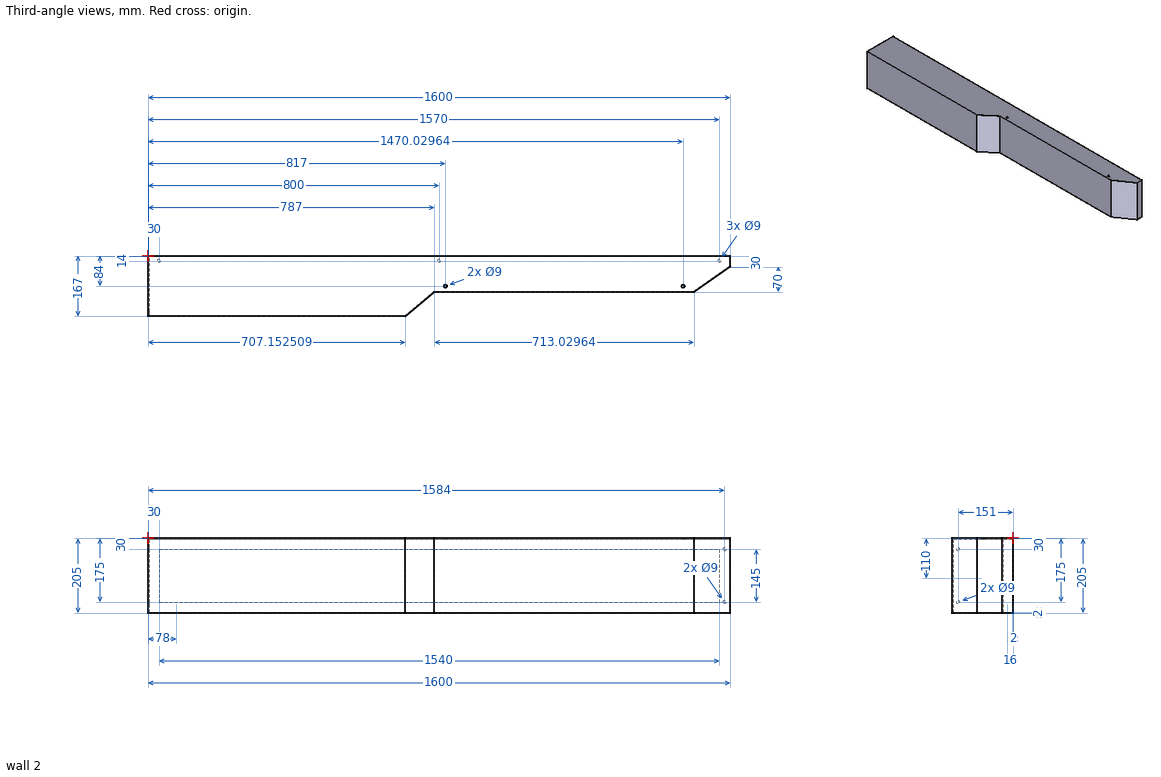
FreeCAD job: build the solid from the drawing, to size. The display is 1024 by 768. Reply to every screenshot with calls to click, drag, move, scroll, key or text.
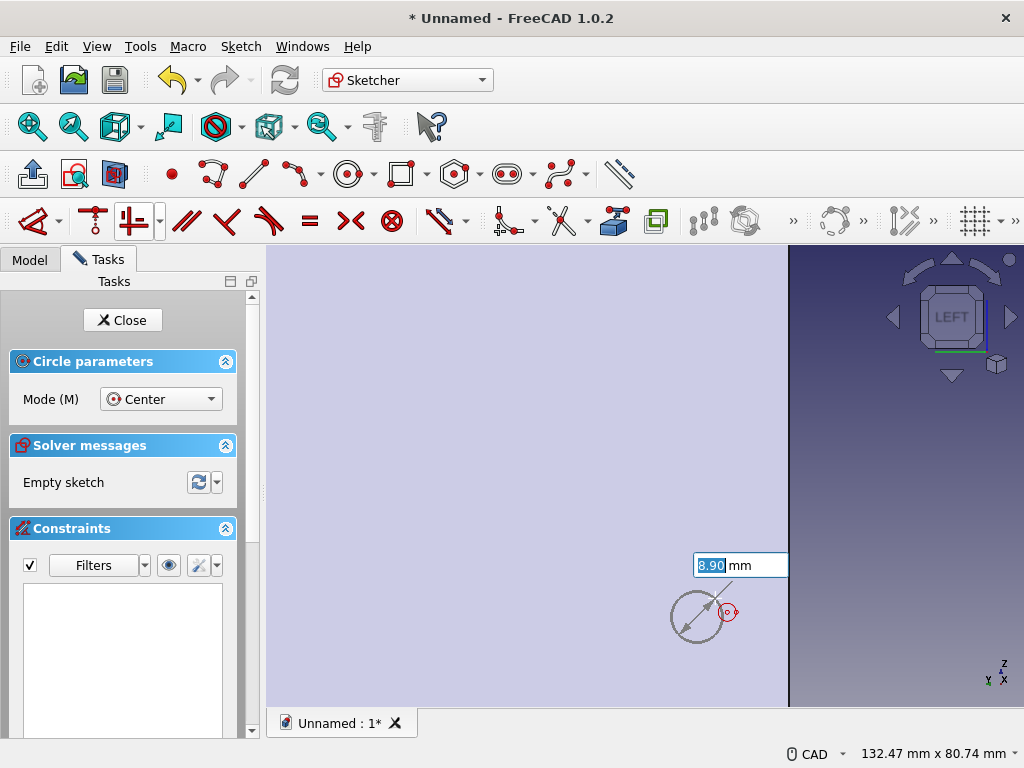
text(9)
key(Return)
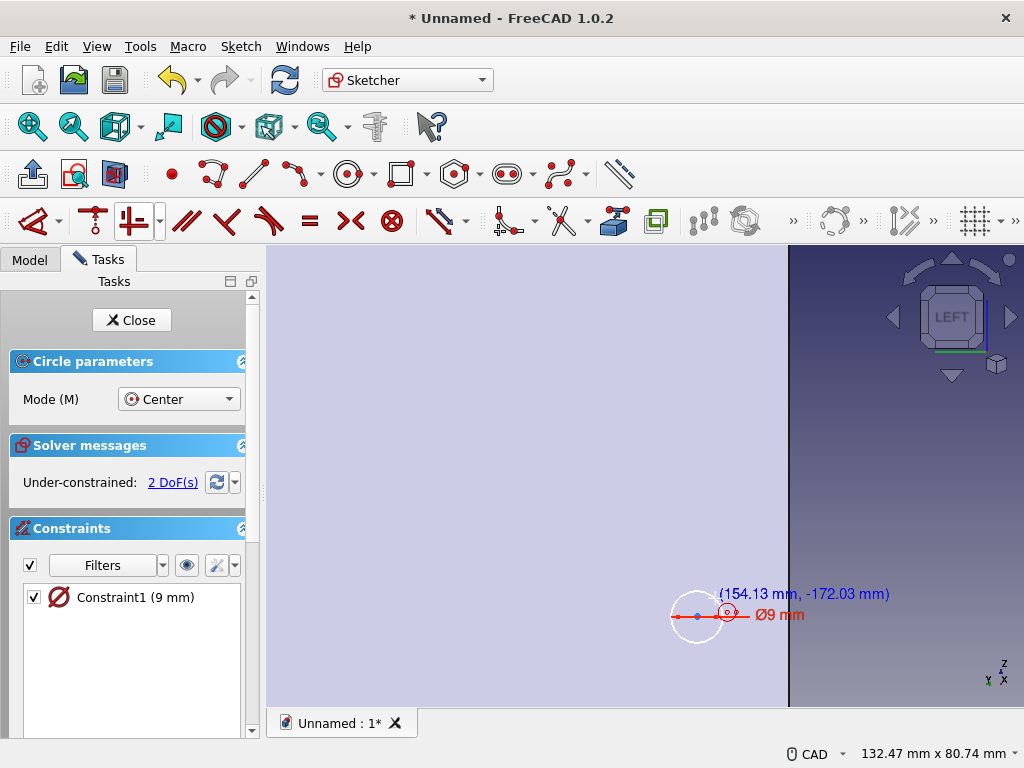
scroll(705, 626, down, 6)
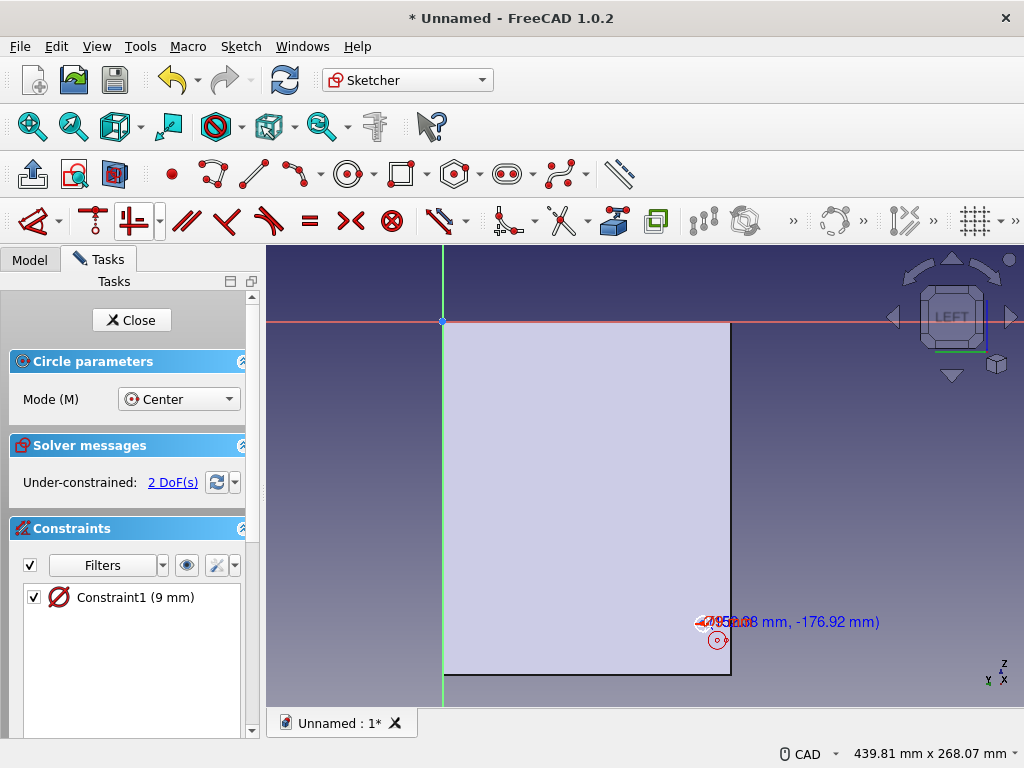
scroll(703, 374, up, 6)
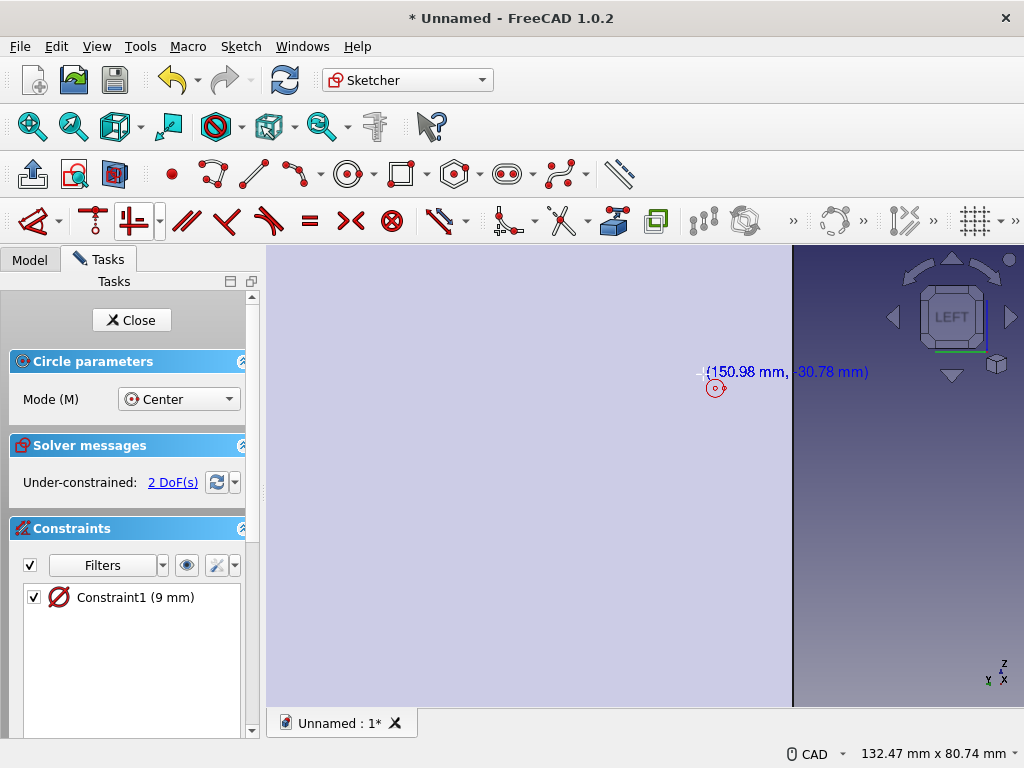
click(702, 372)
move(720, 354)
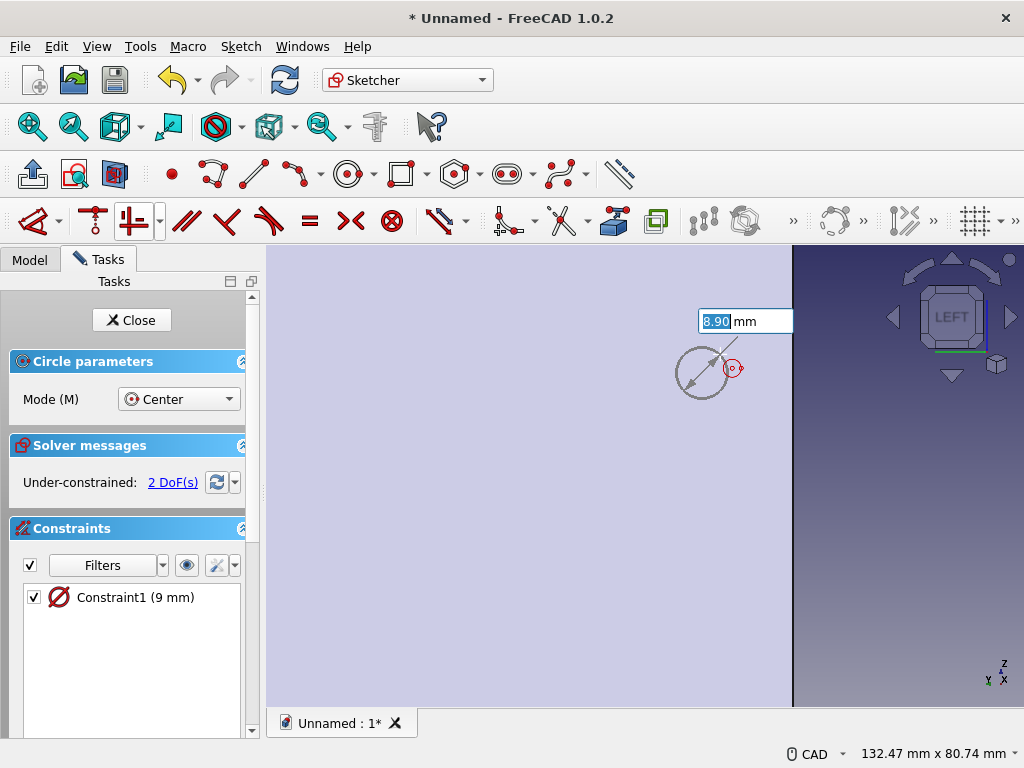
text(9)
key(Return)
key(Escape)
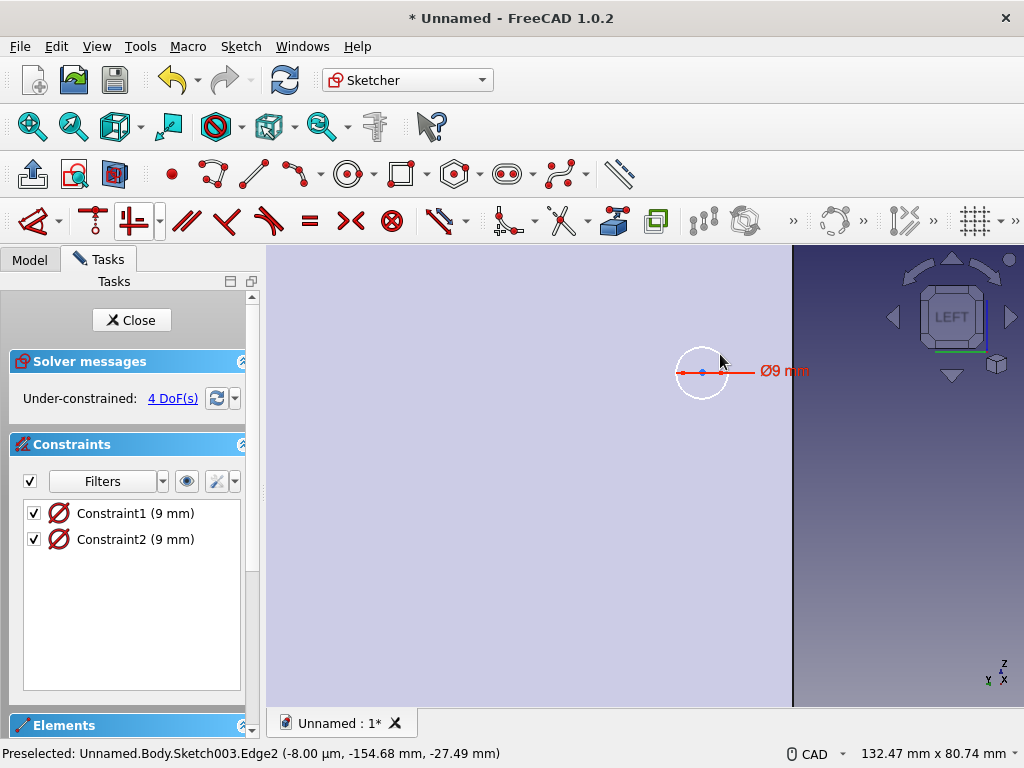
key(d)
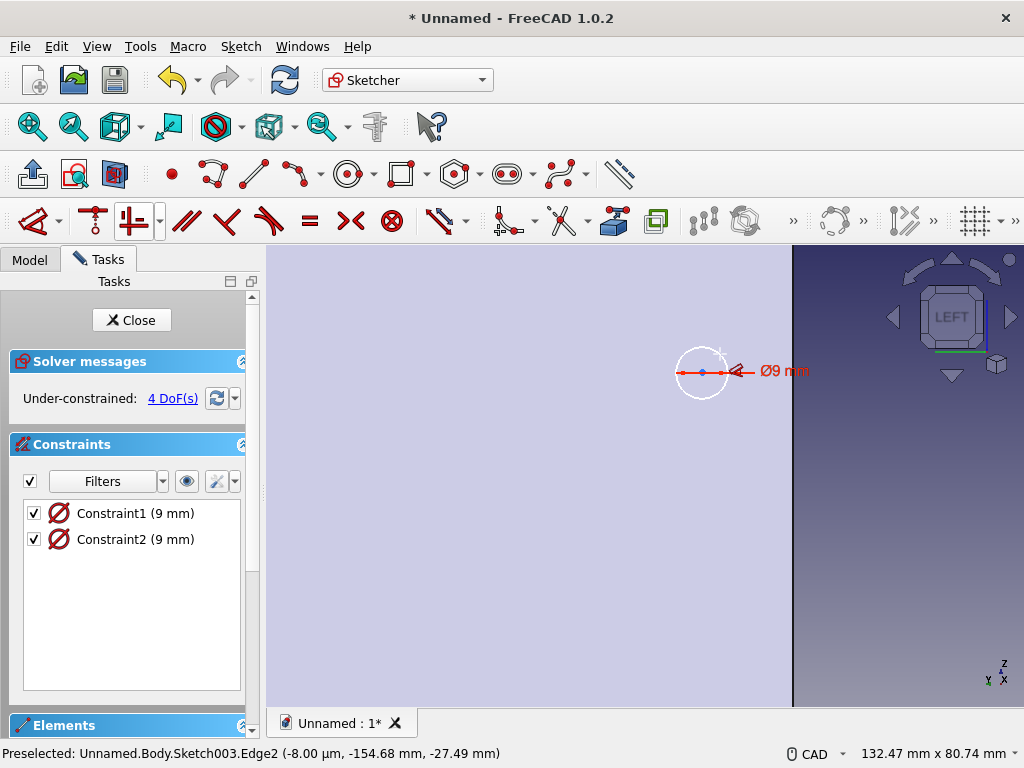
click(702, 373)
click(736, 323)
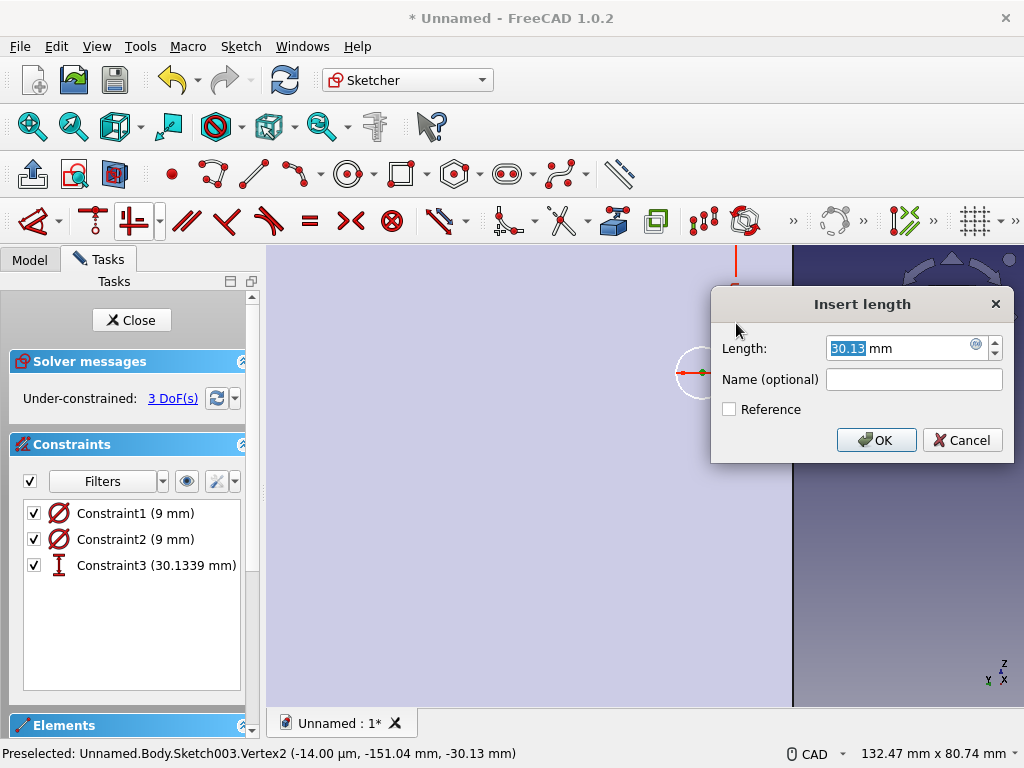
text(30)
key(Return)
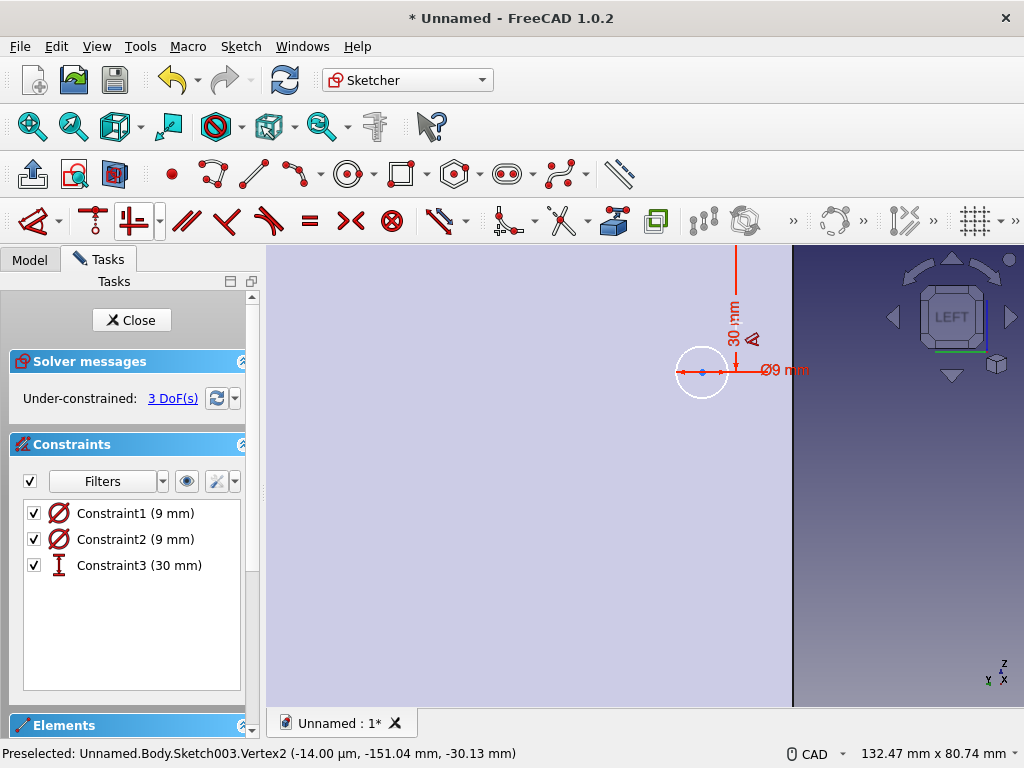
scroll(703, 373, down, 6)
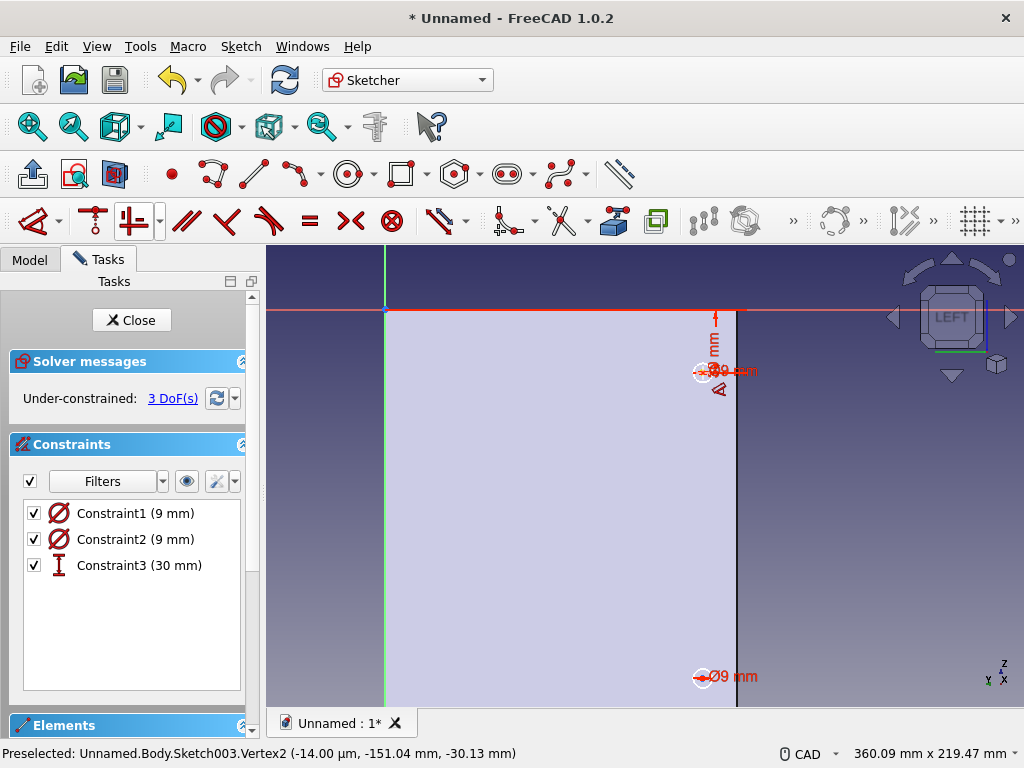
click(703, 623)
click(573, 287)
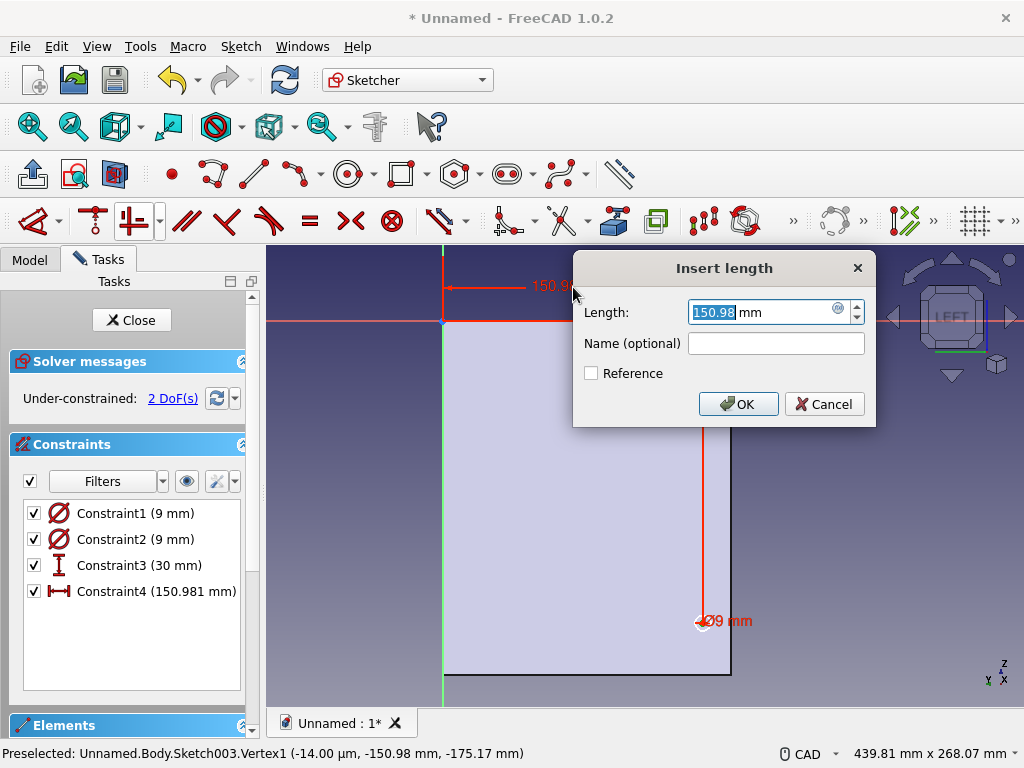
text(151)
key(Return)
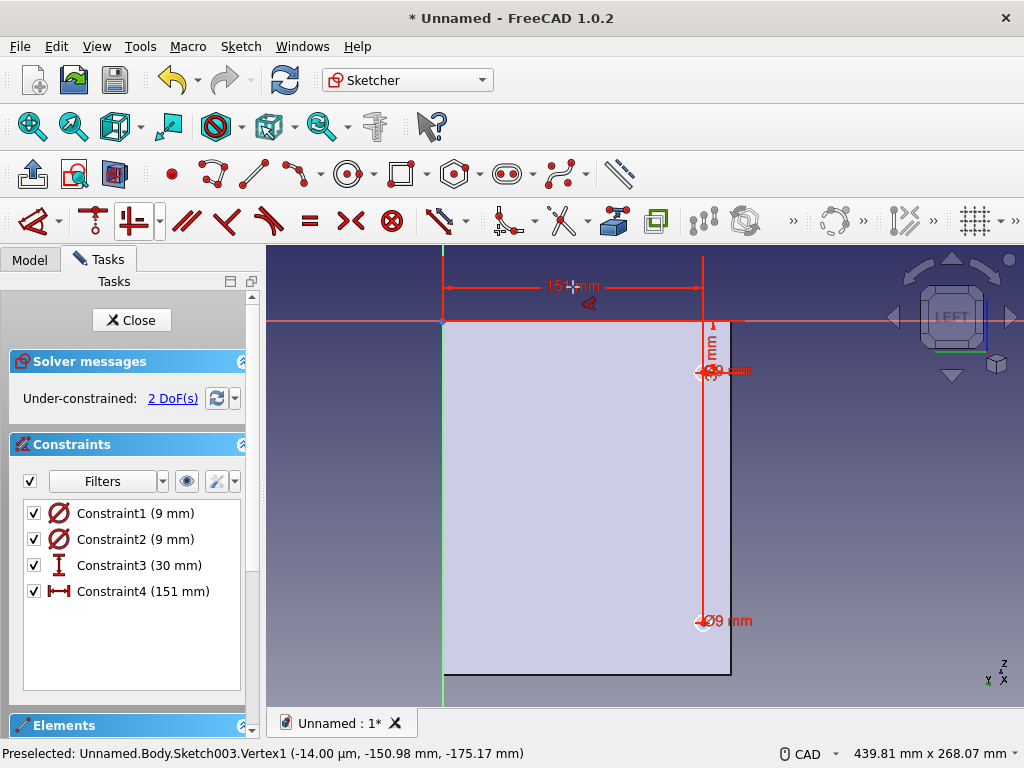
click(703, 623)
click(409, 472)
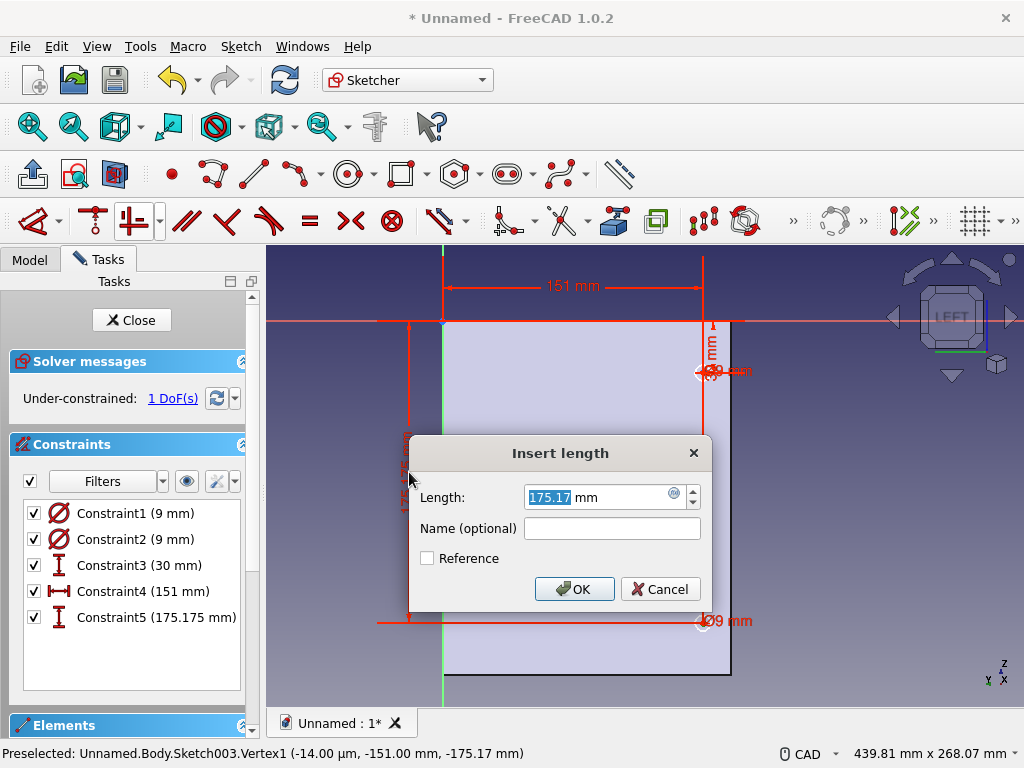
text(175)
key(Return)